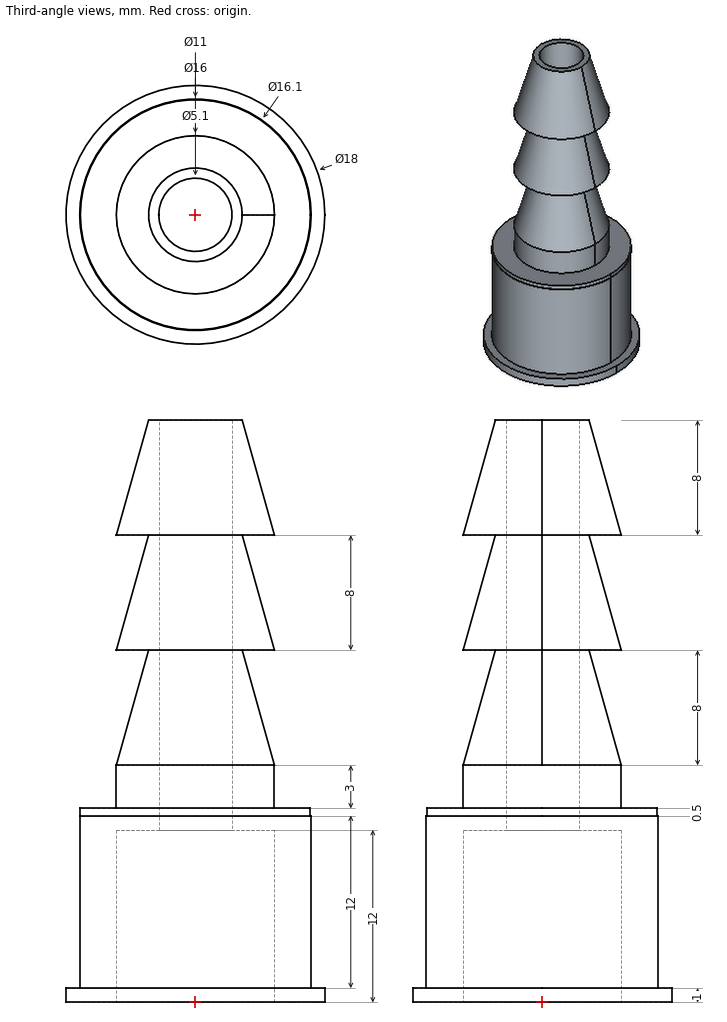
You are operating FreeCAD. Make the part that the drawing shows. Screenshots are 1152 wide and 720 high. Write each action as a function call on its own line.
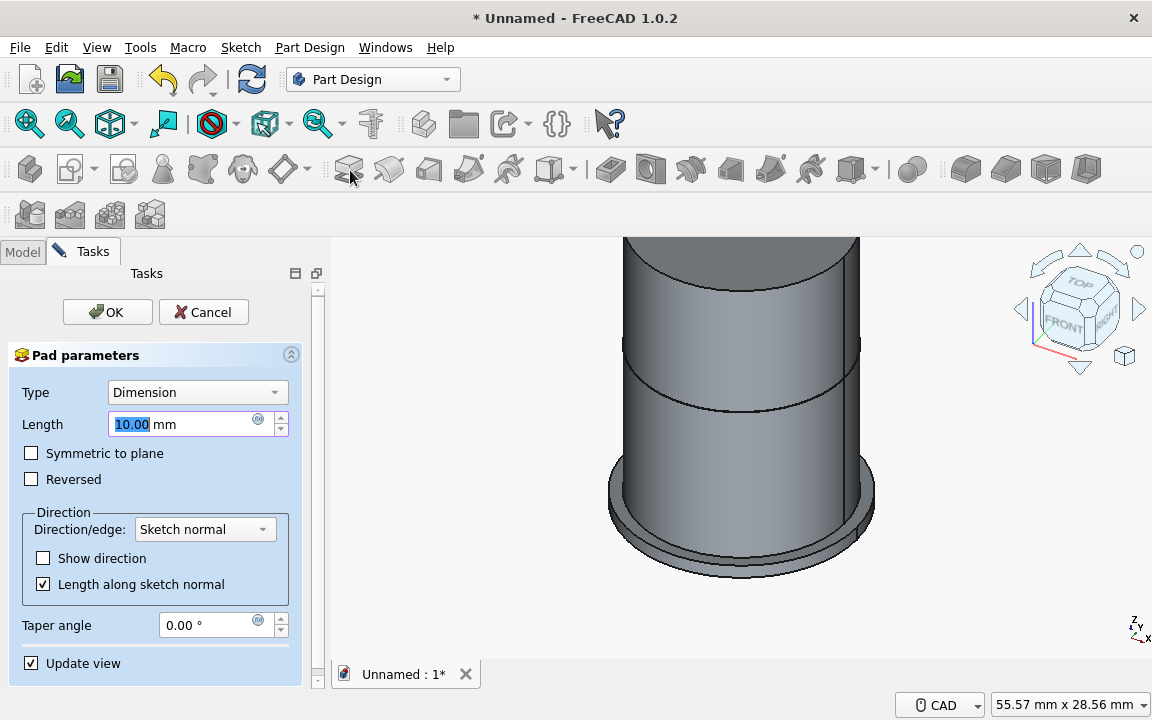
text(0.5)
key(Tab)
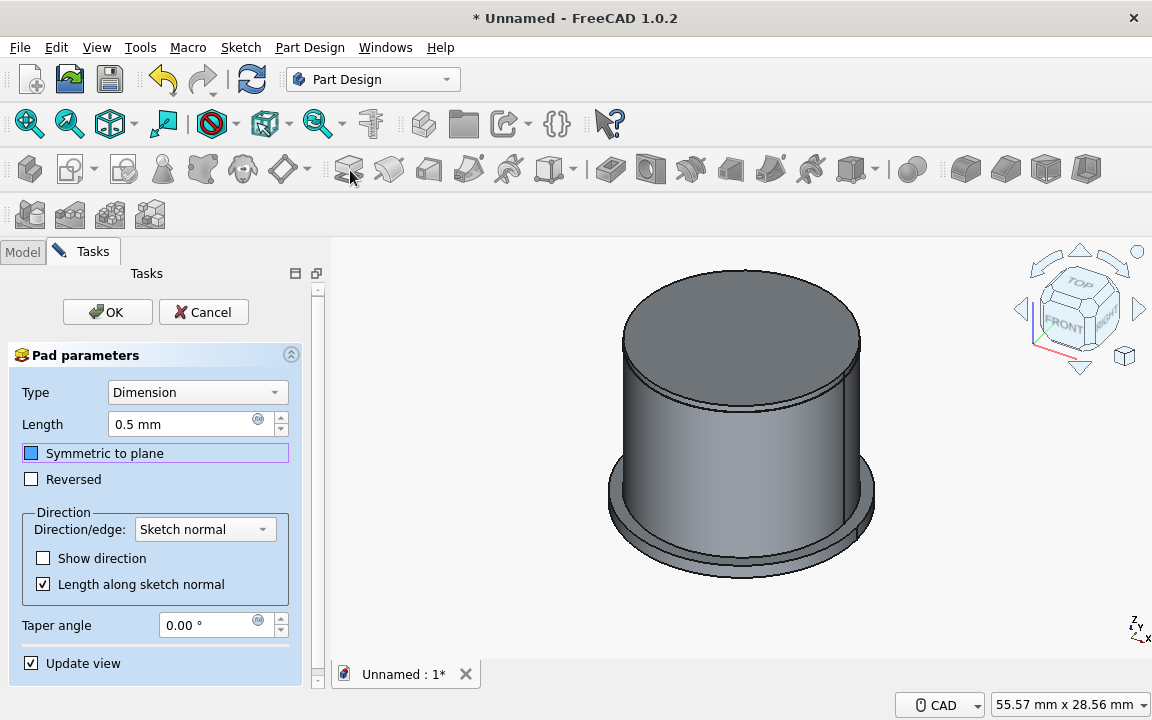
click(108, 312)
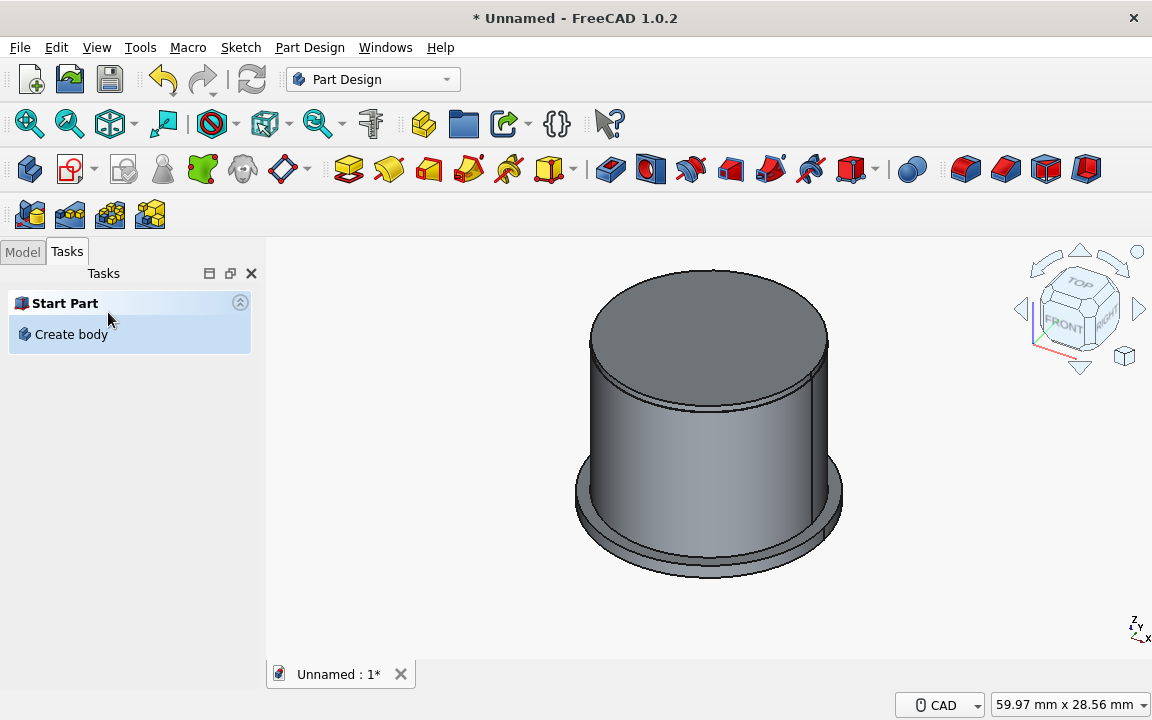
key(v)
key(f)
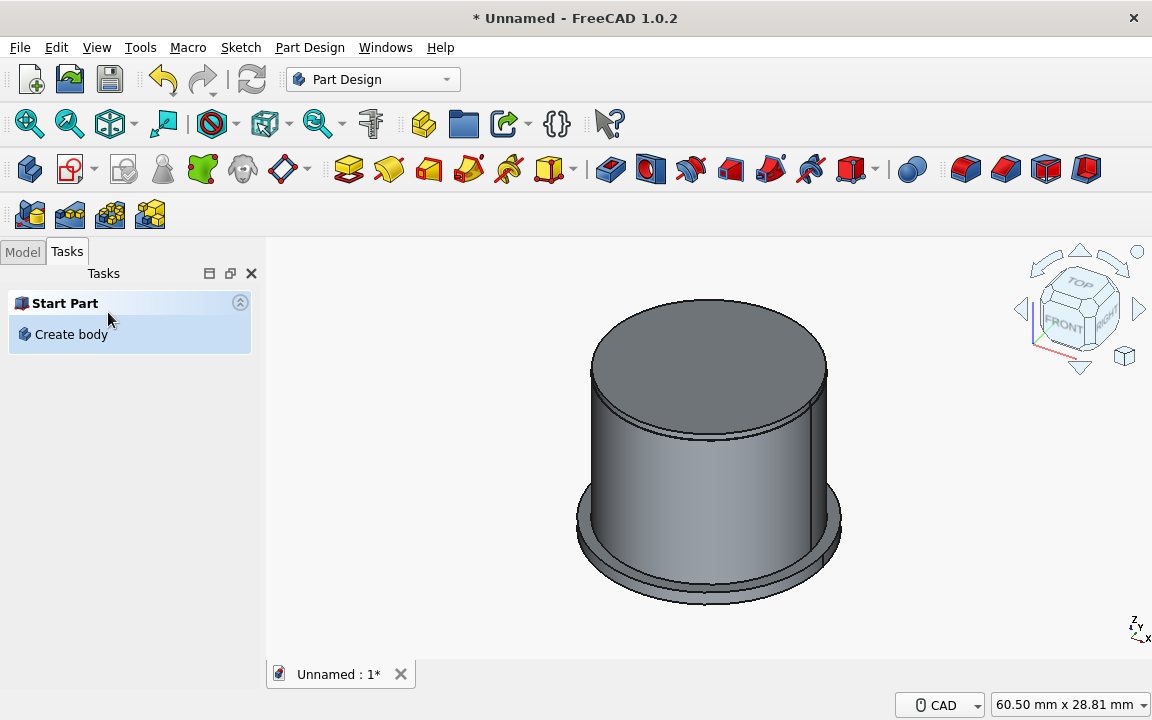
click(709, 366)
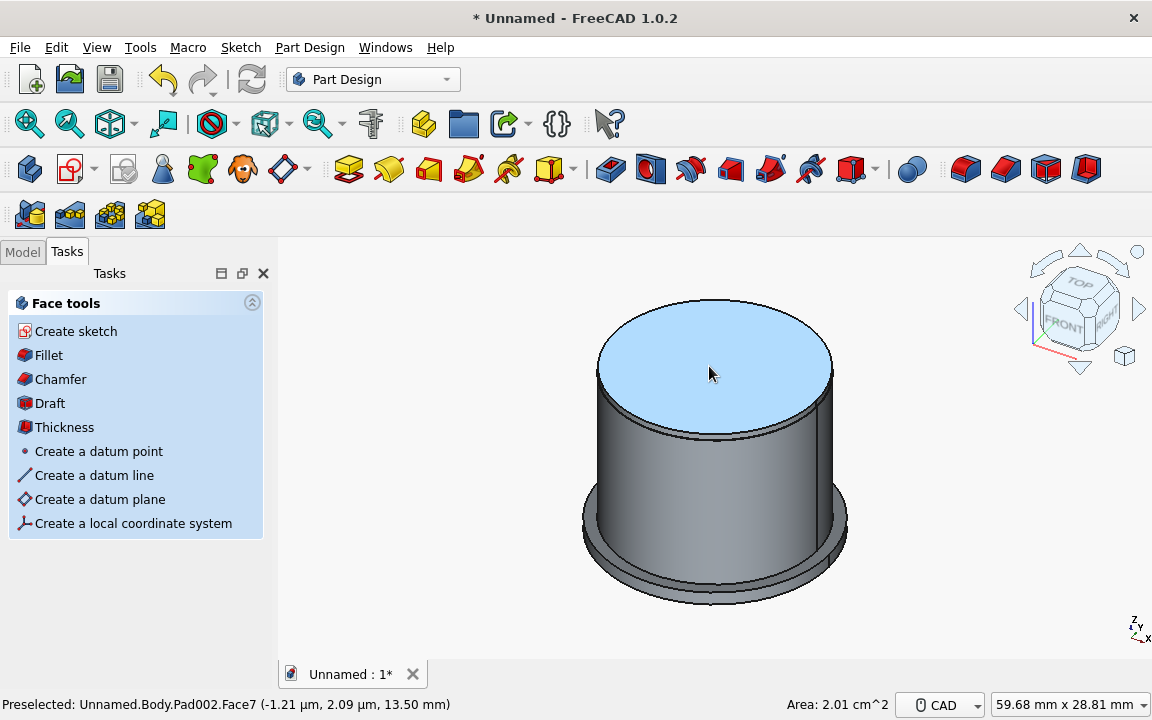
click(70, 170)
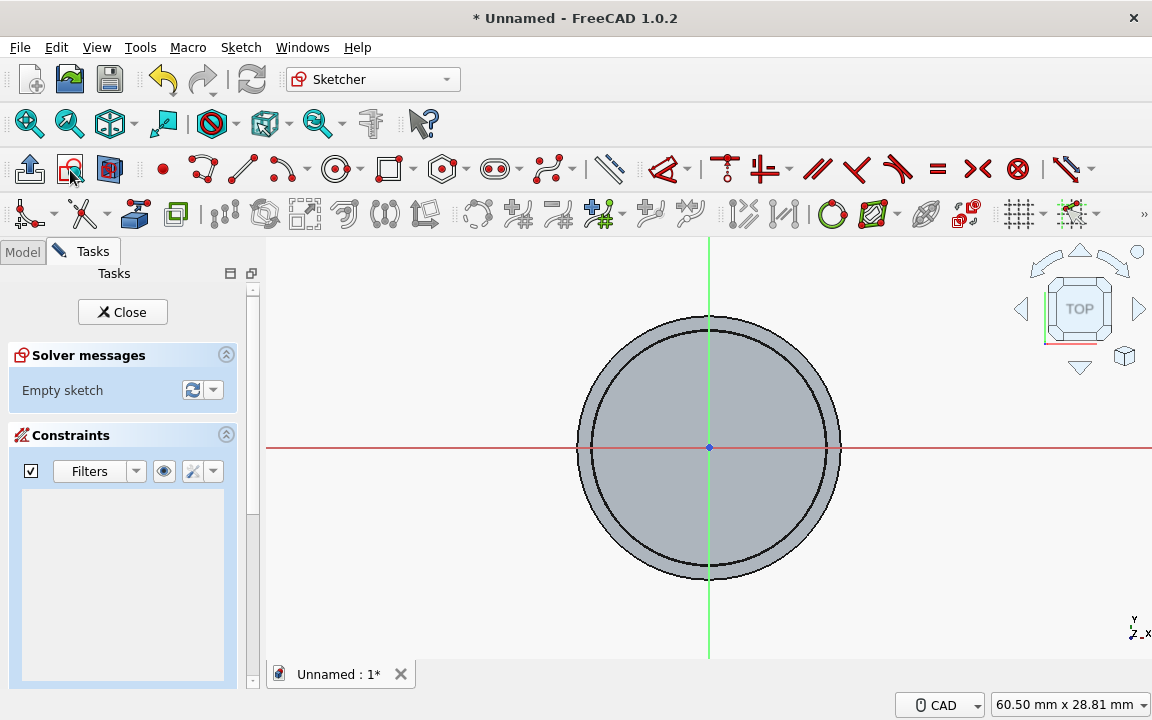
scroll(848, 448, up, 2)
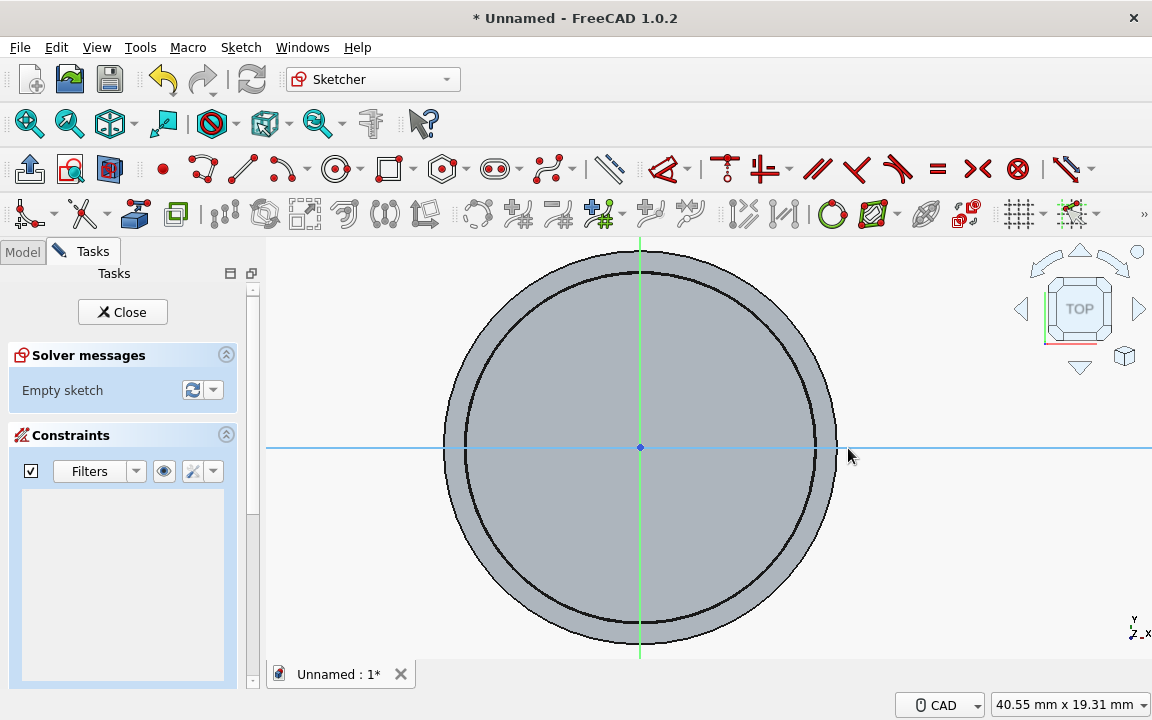
click(336, 170)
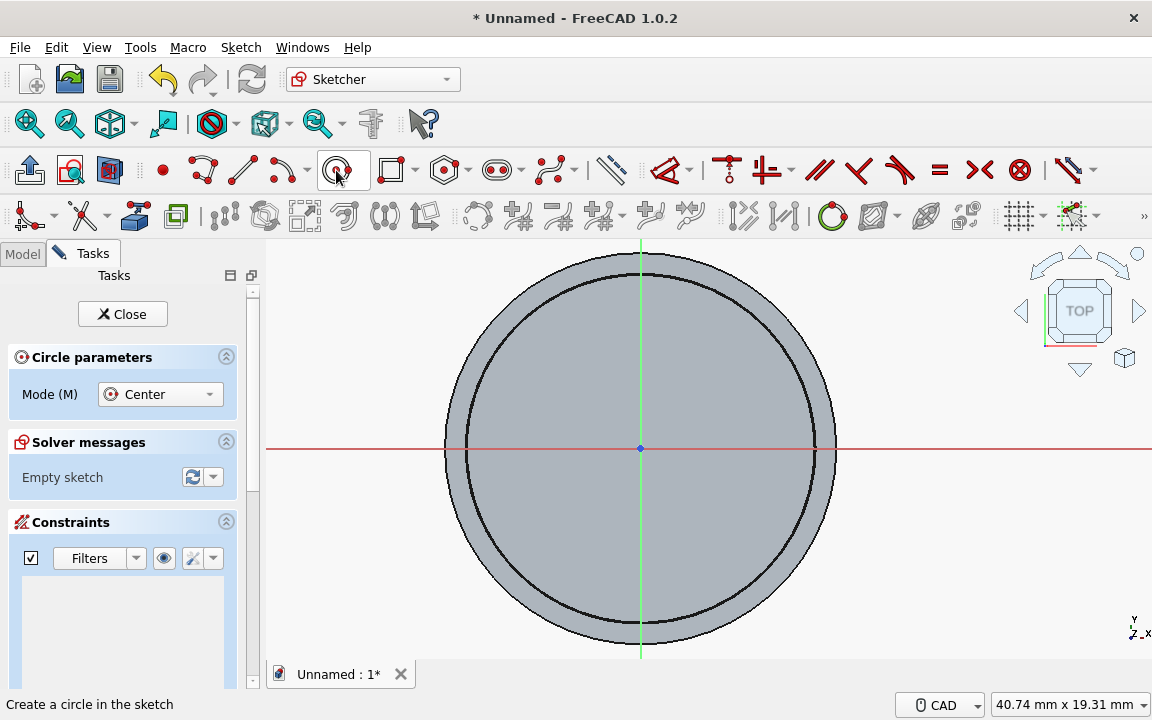
click(641, 449)
click(725, 364)
key(Escape)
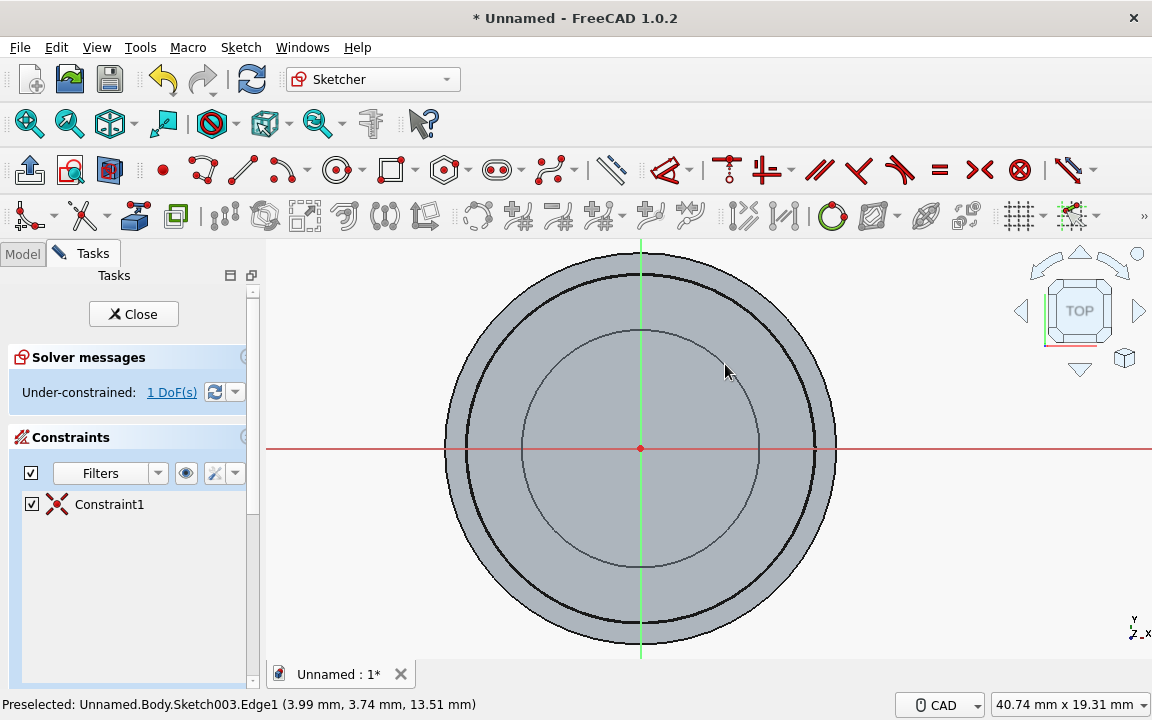
key(d)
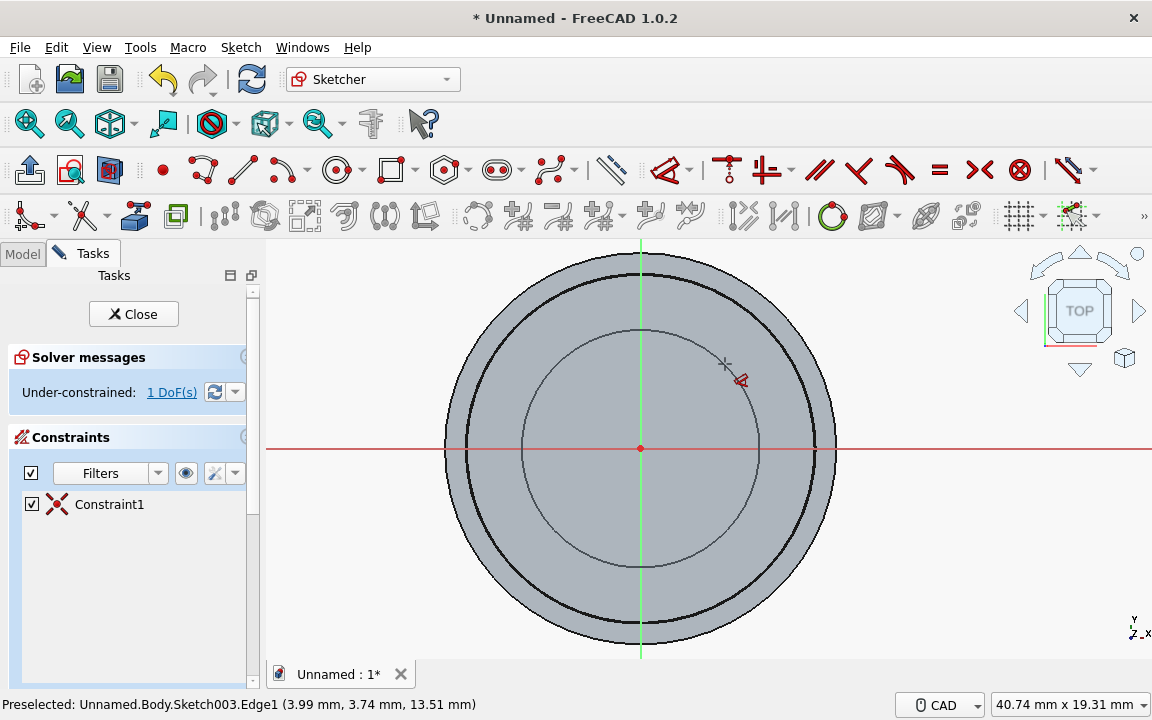
click(724, 364)
click(746, 341)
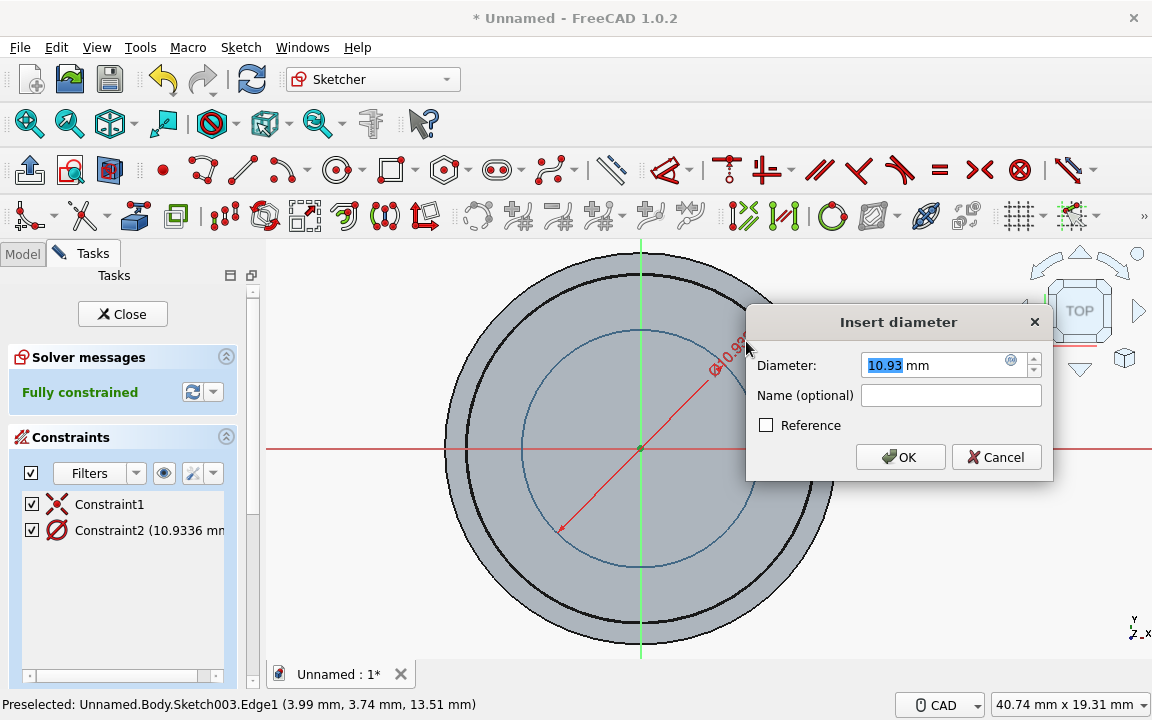
text(11)
key(Return)
key(Escape)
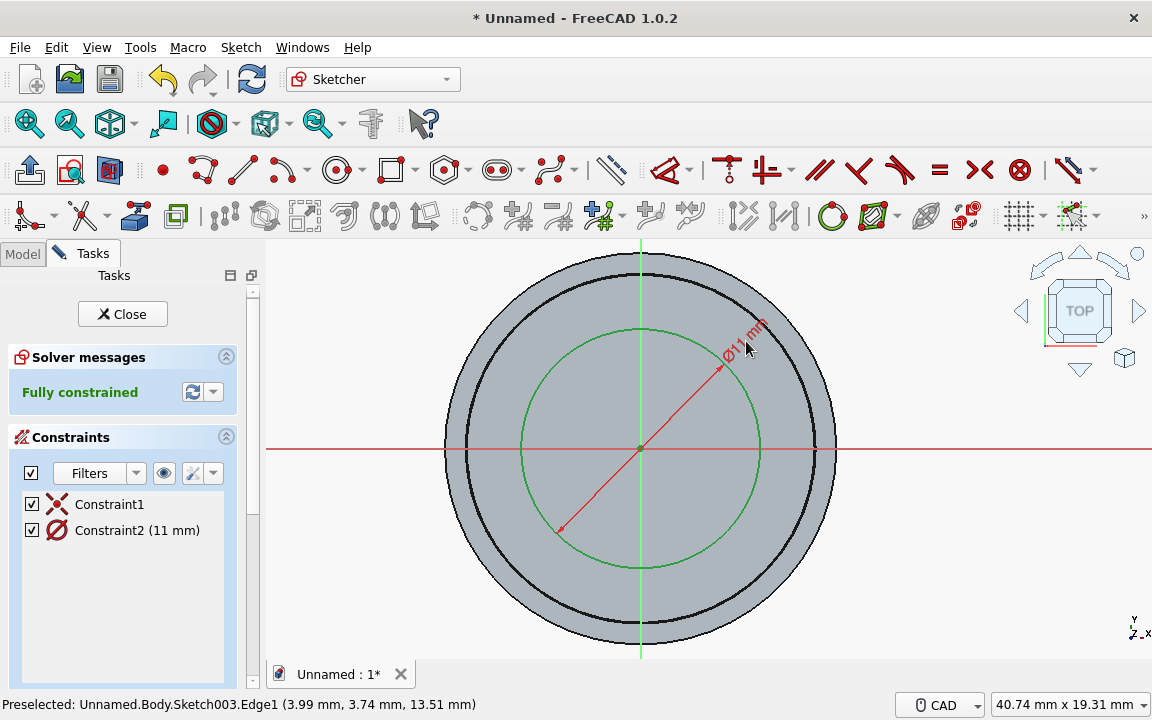
click(123, 314)